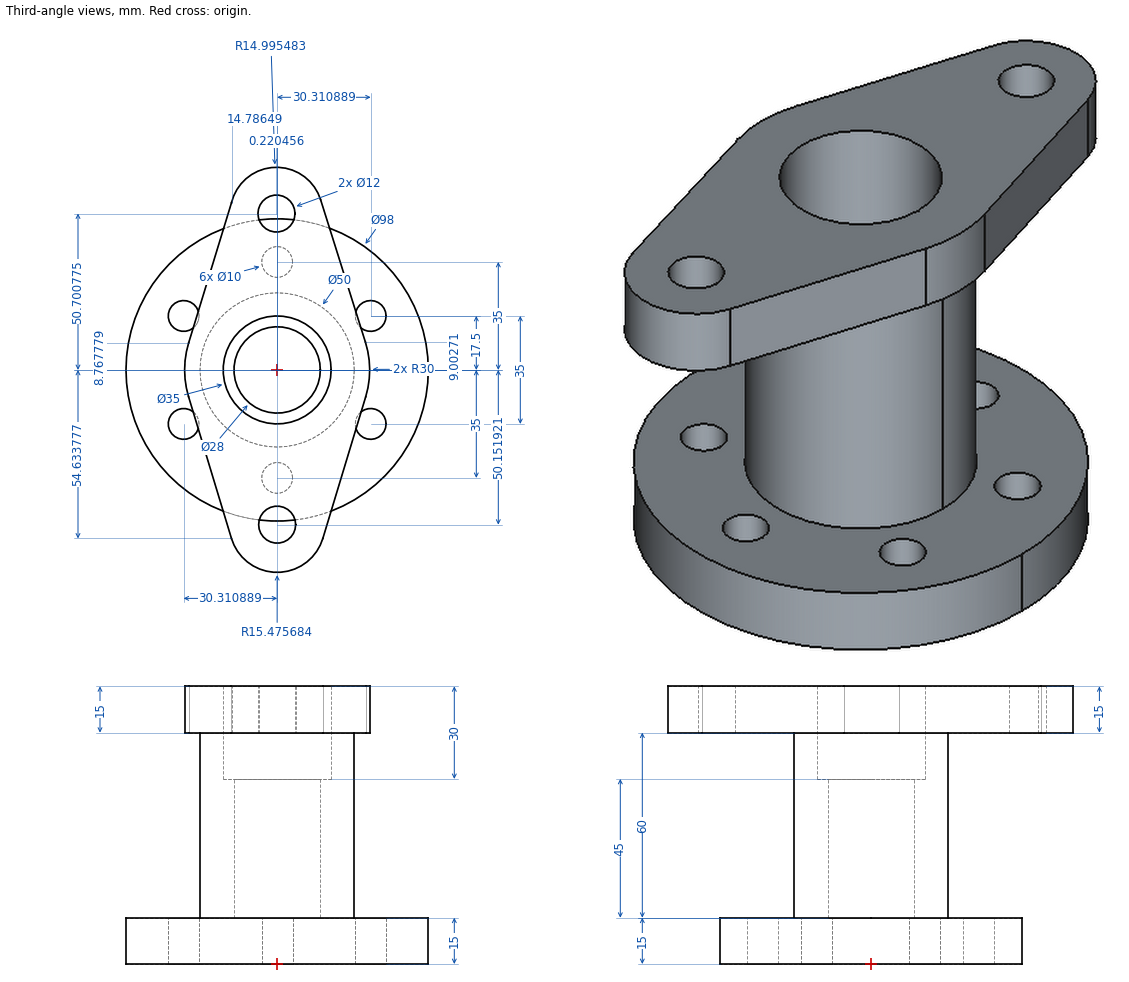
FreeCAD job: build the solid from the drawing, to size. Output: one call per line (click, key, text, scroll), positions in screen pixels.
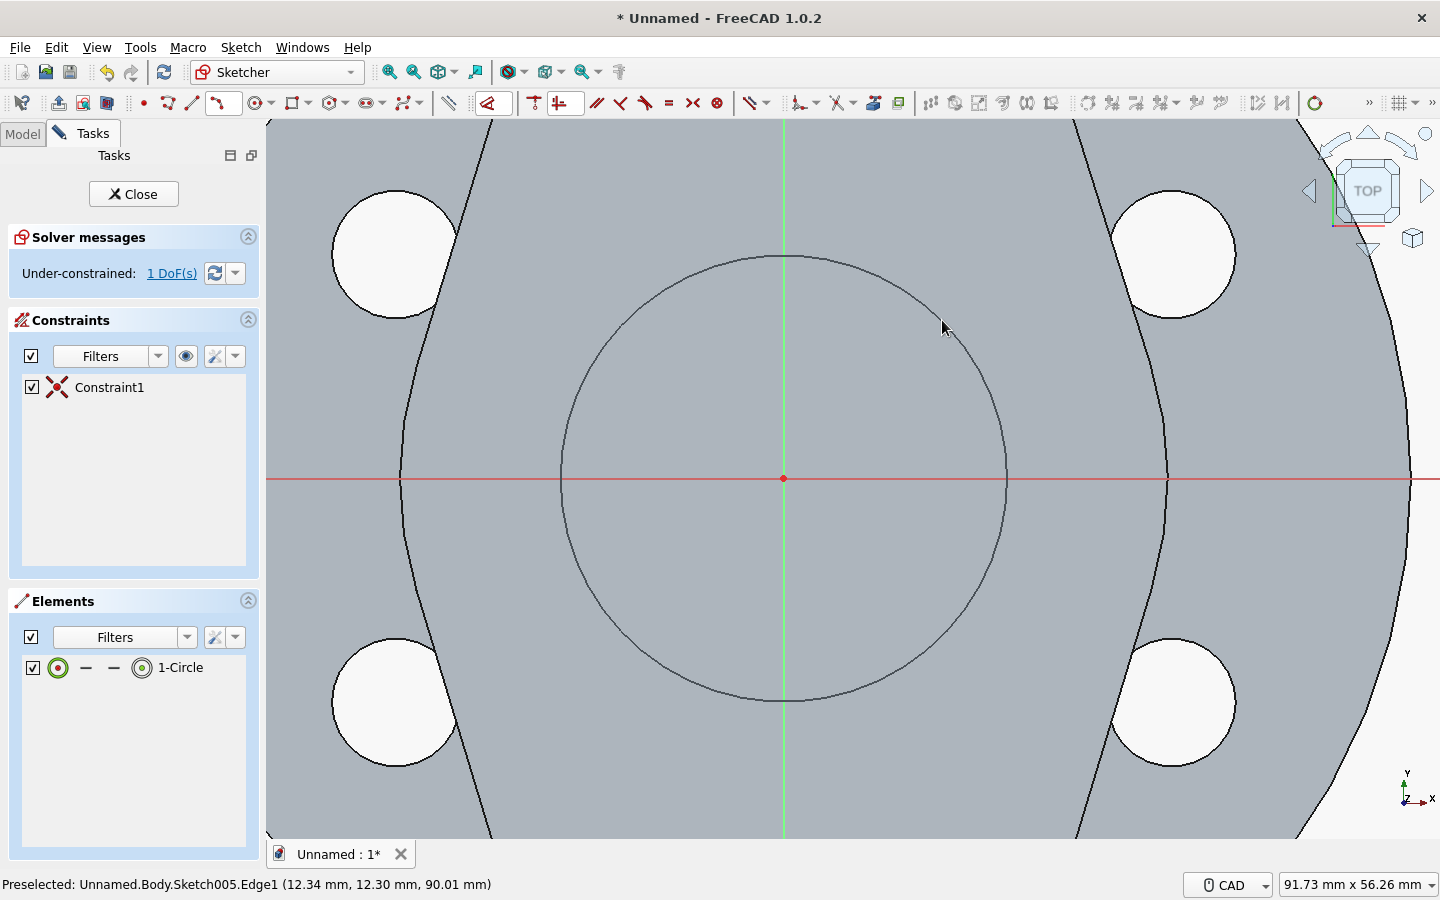
click(941, 320)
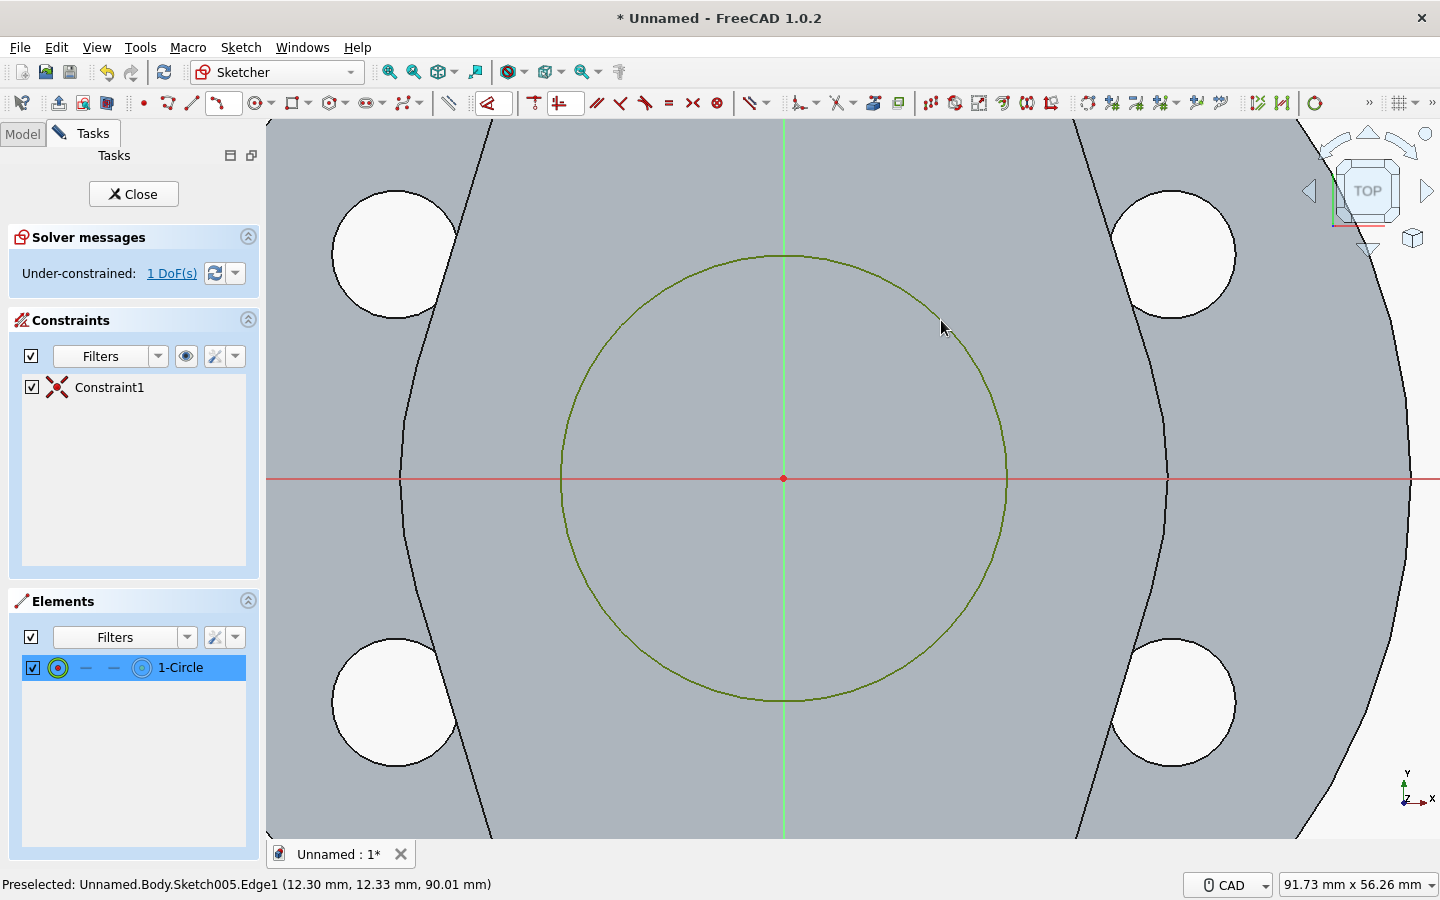
key(k)
key(o)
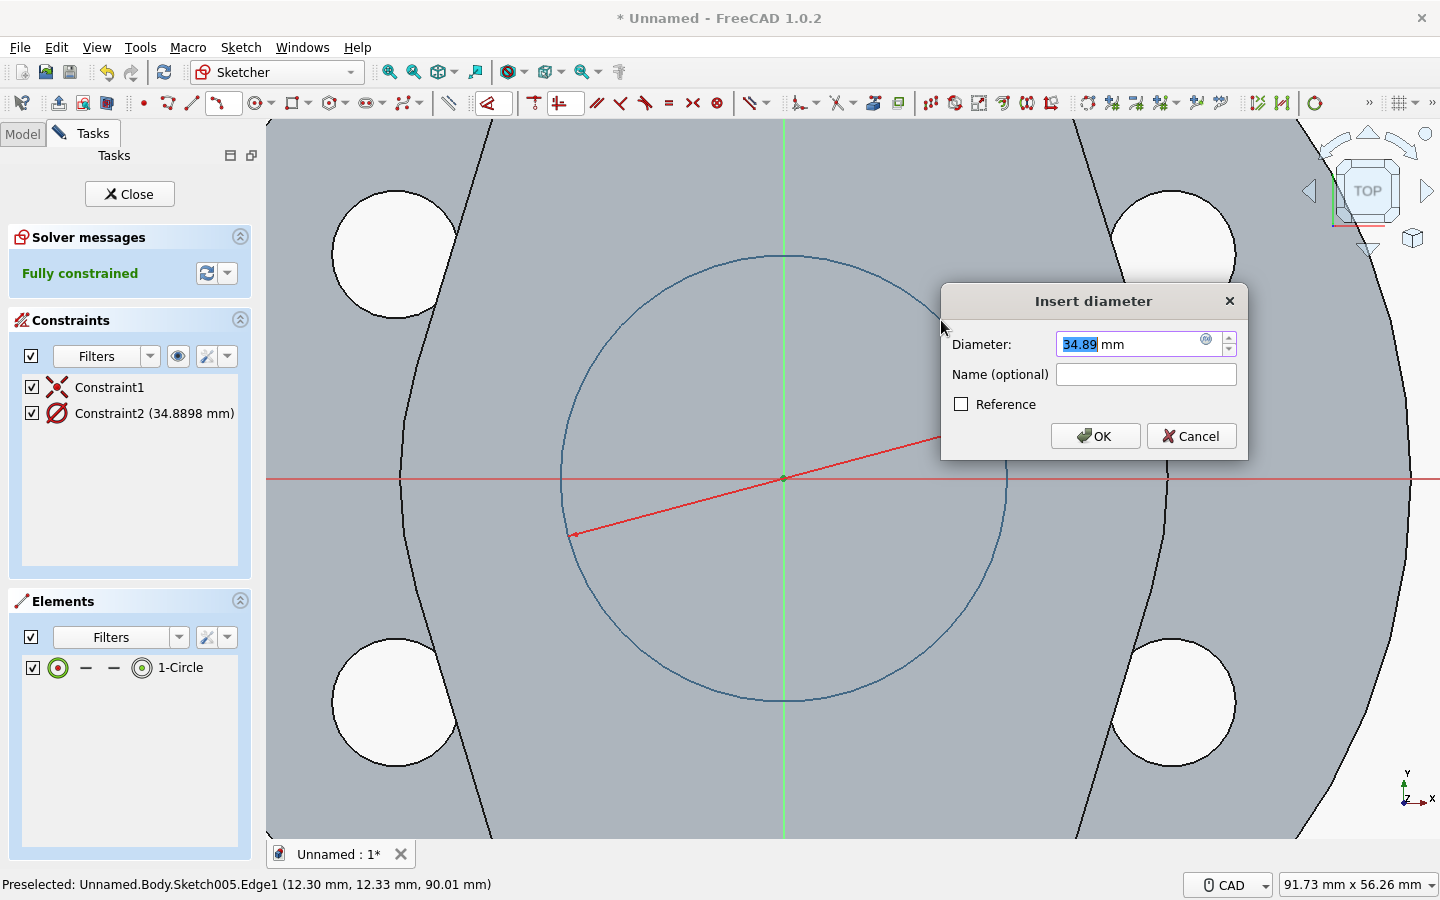
text(35)
key(Return)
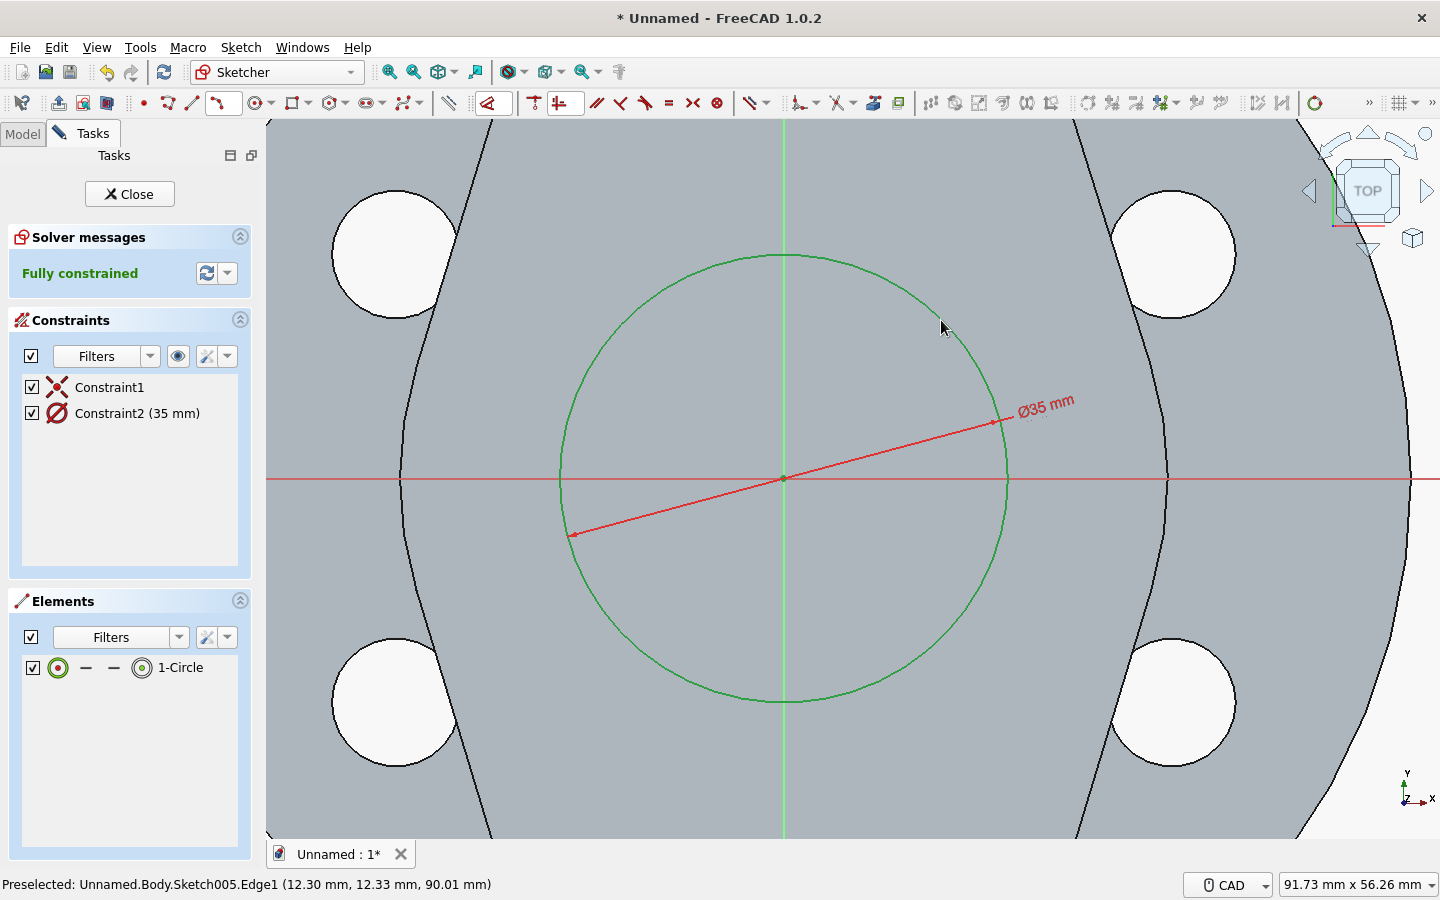
click(130, 194)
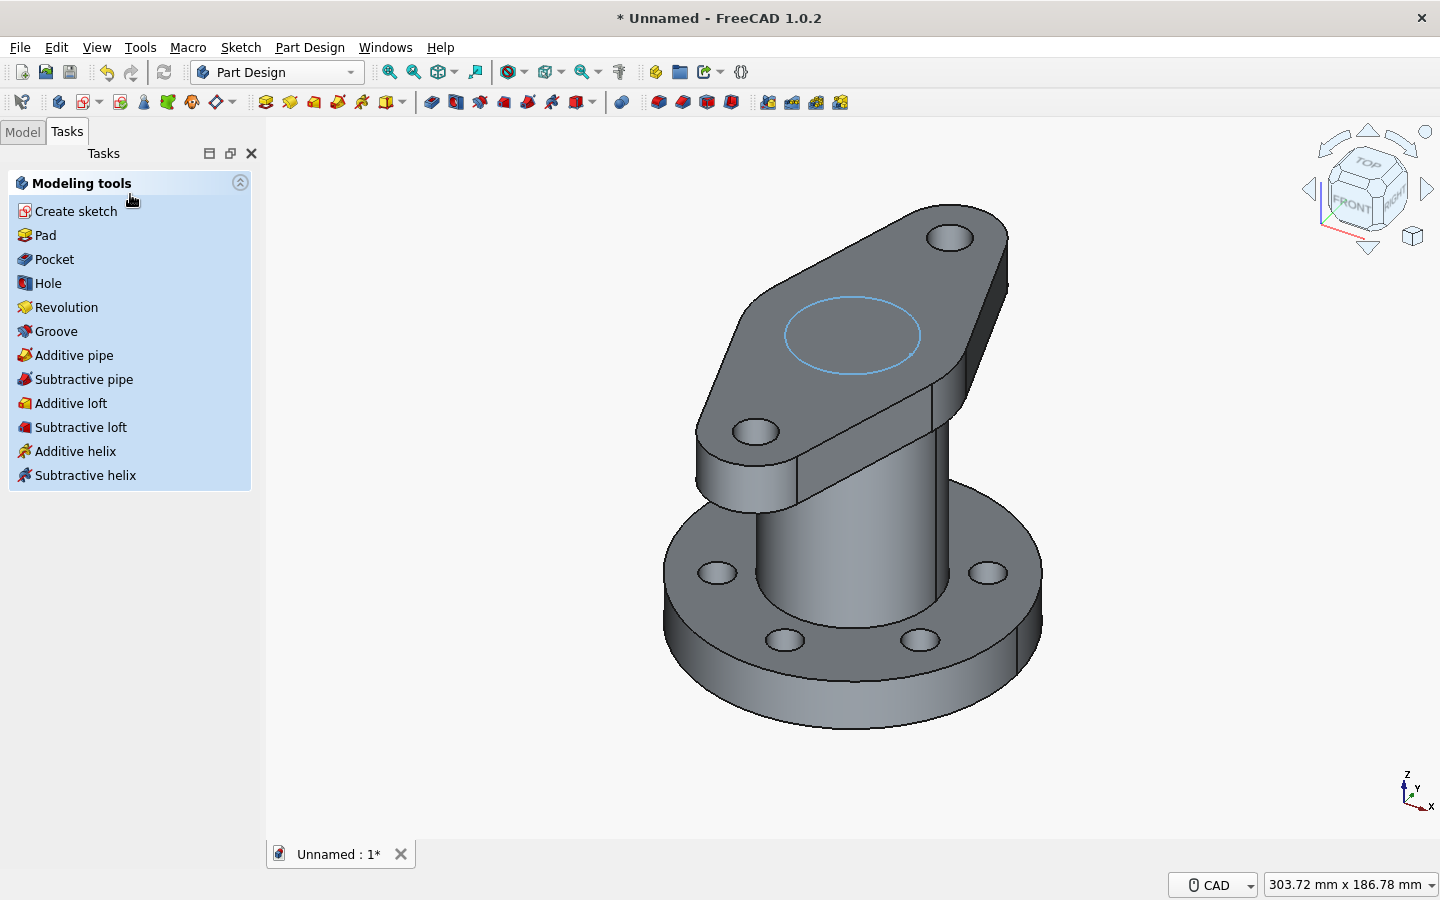
click(432, 102)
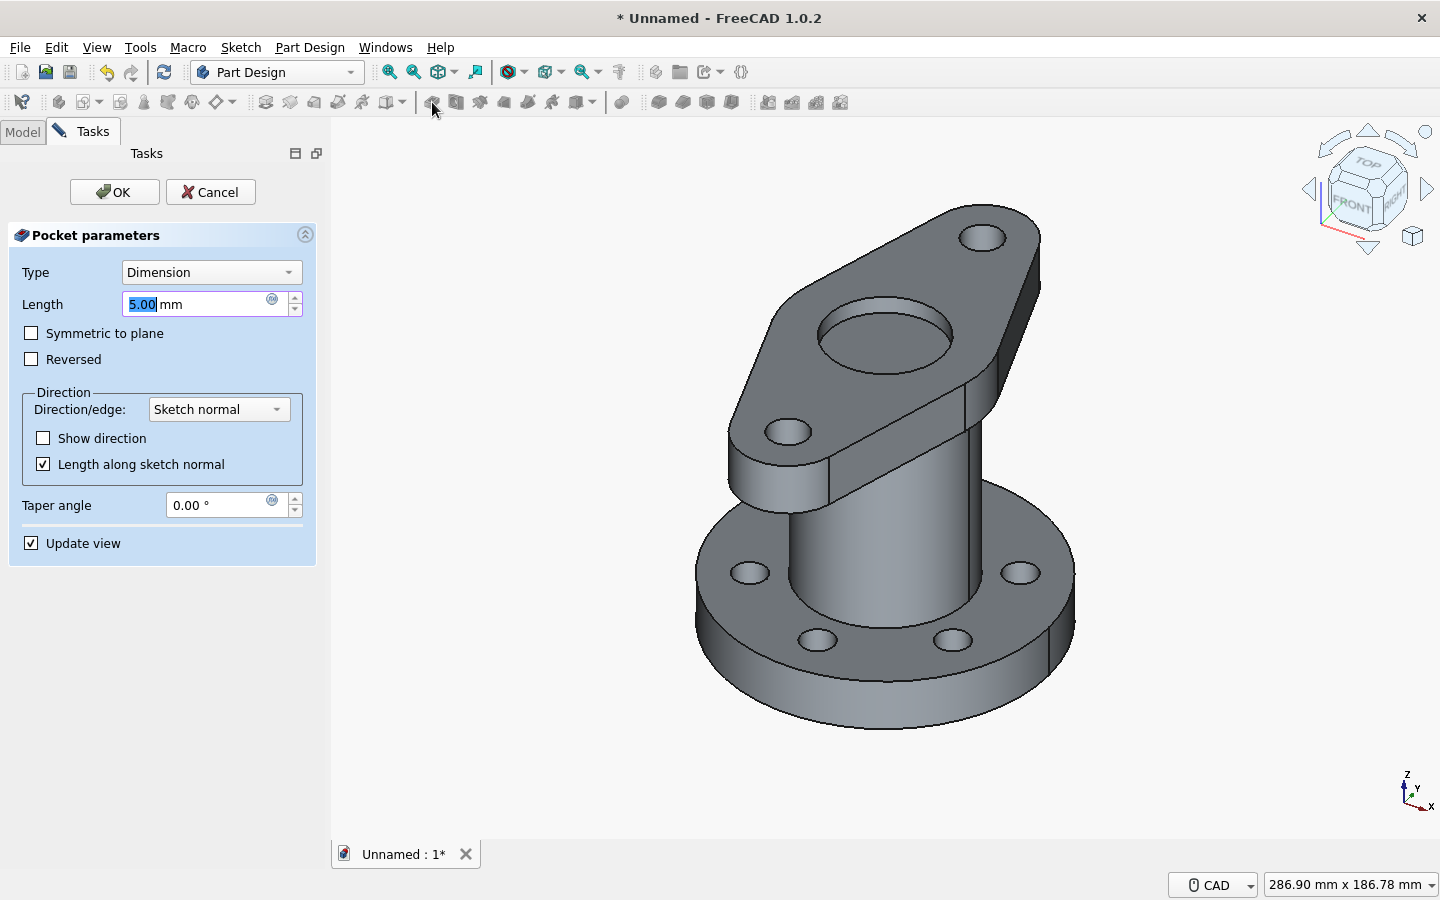
text(30)
key(Tab)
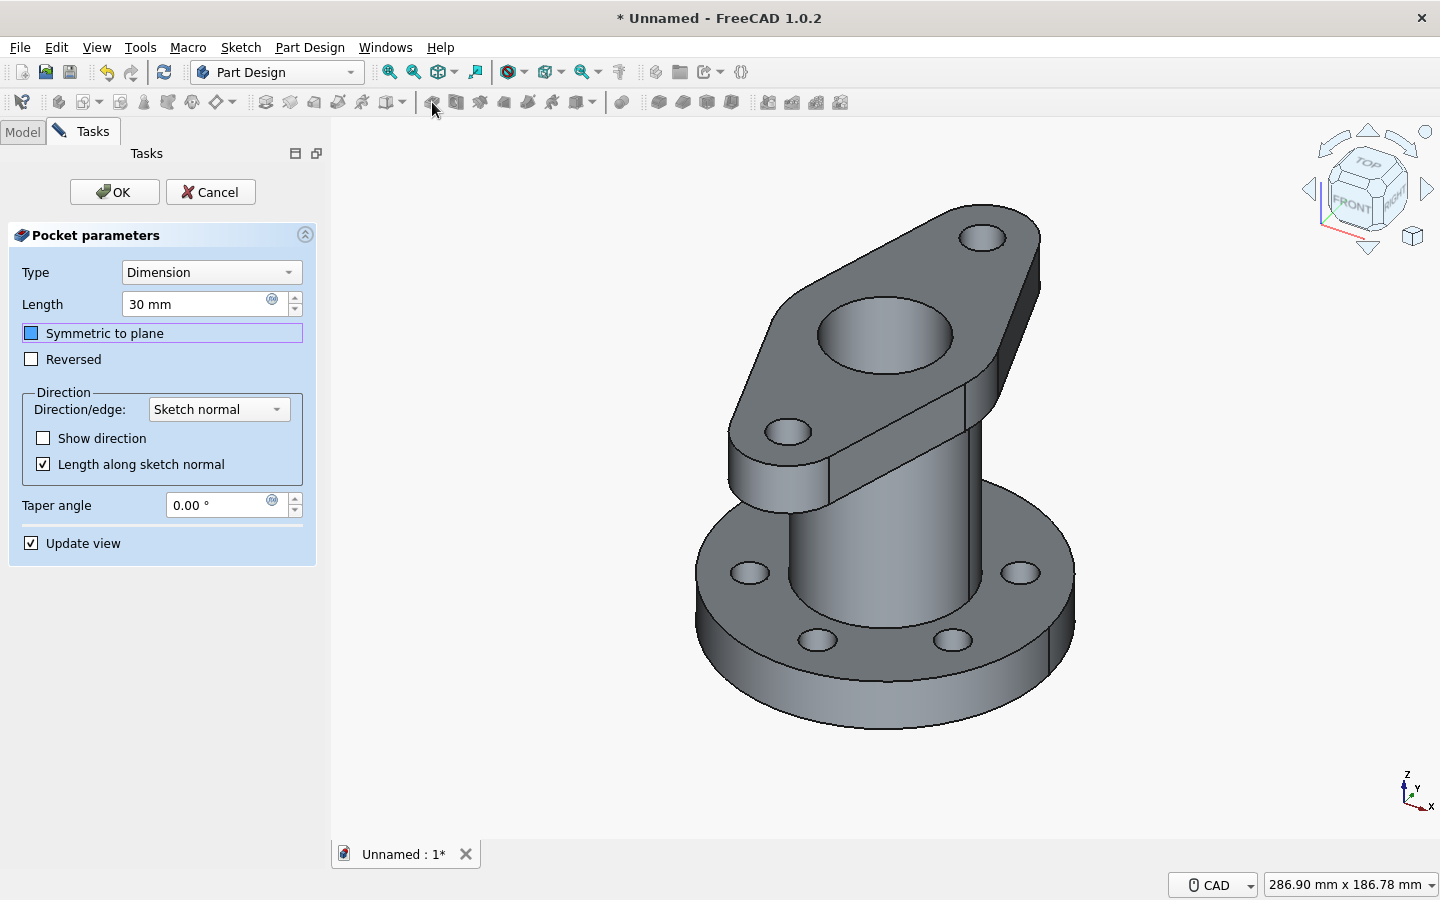
click(115, 192)